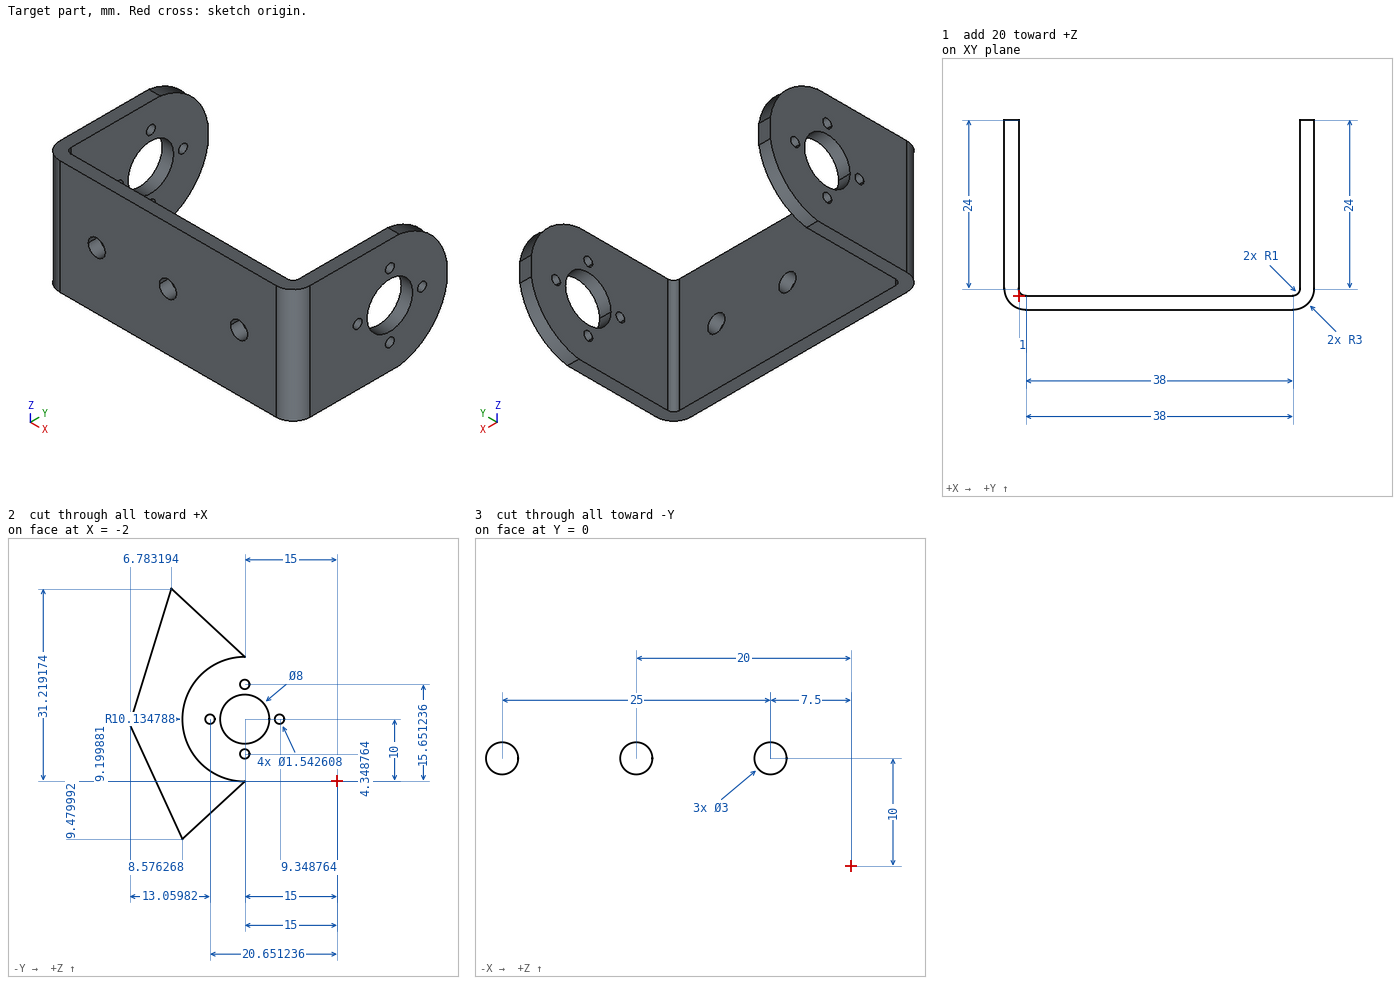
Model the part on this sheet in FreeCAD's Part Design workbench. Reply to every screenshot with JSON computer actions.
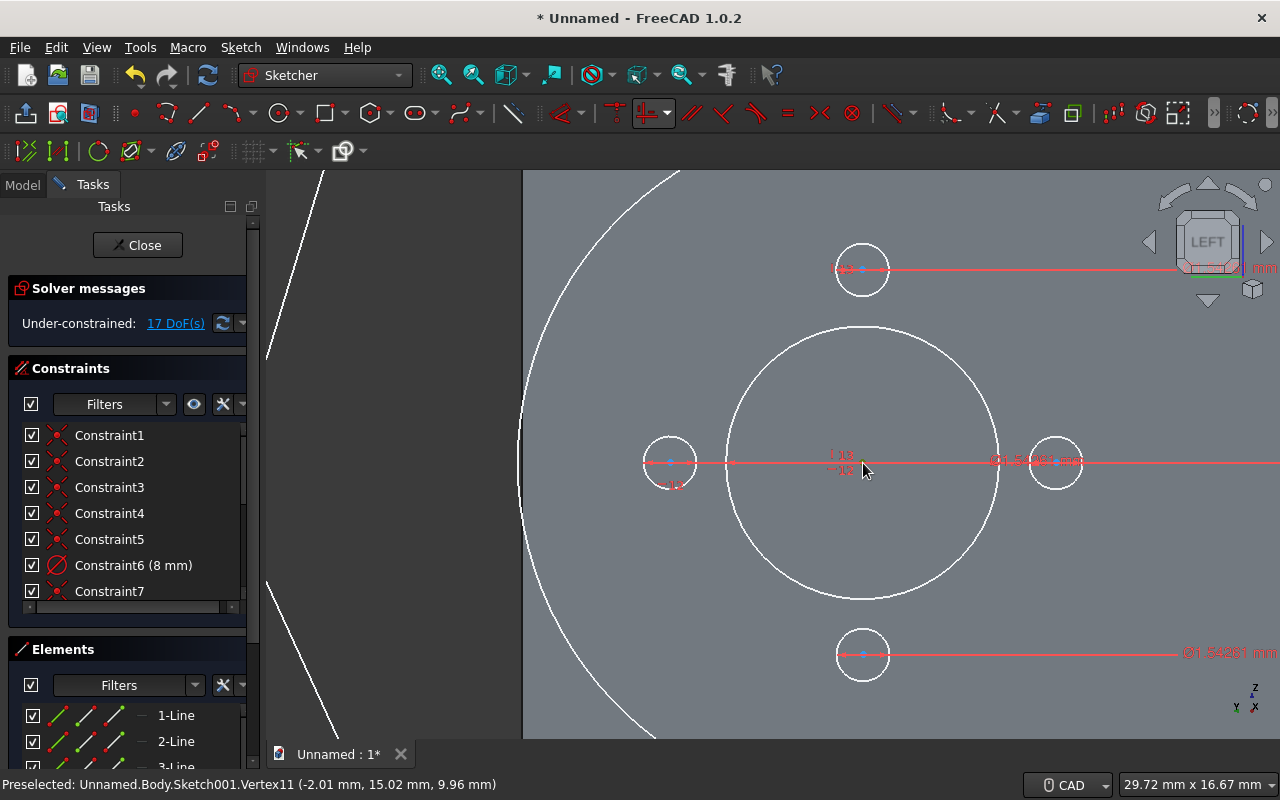
{"action": "left_click", "coordinate": [1056, 463]}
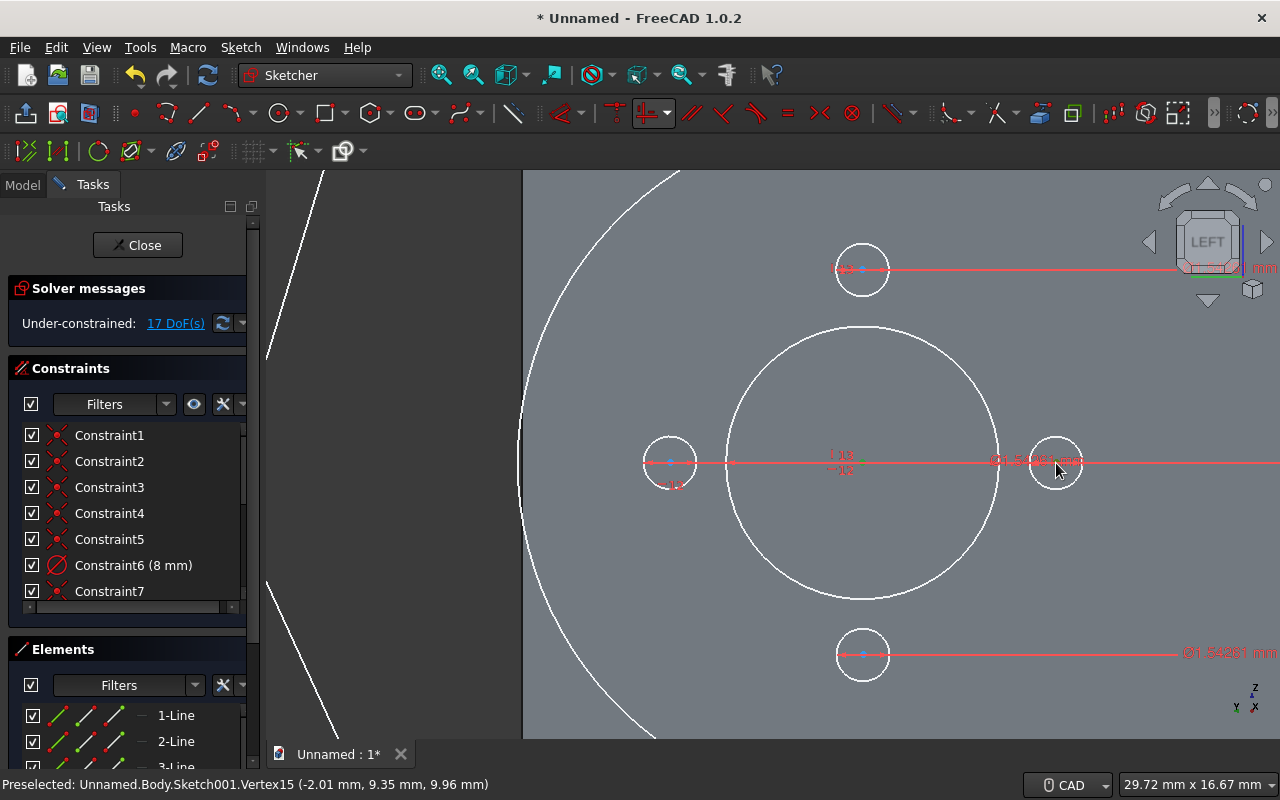
{"action": "left_click", "coordinate": [670, 114]}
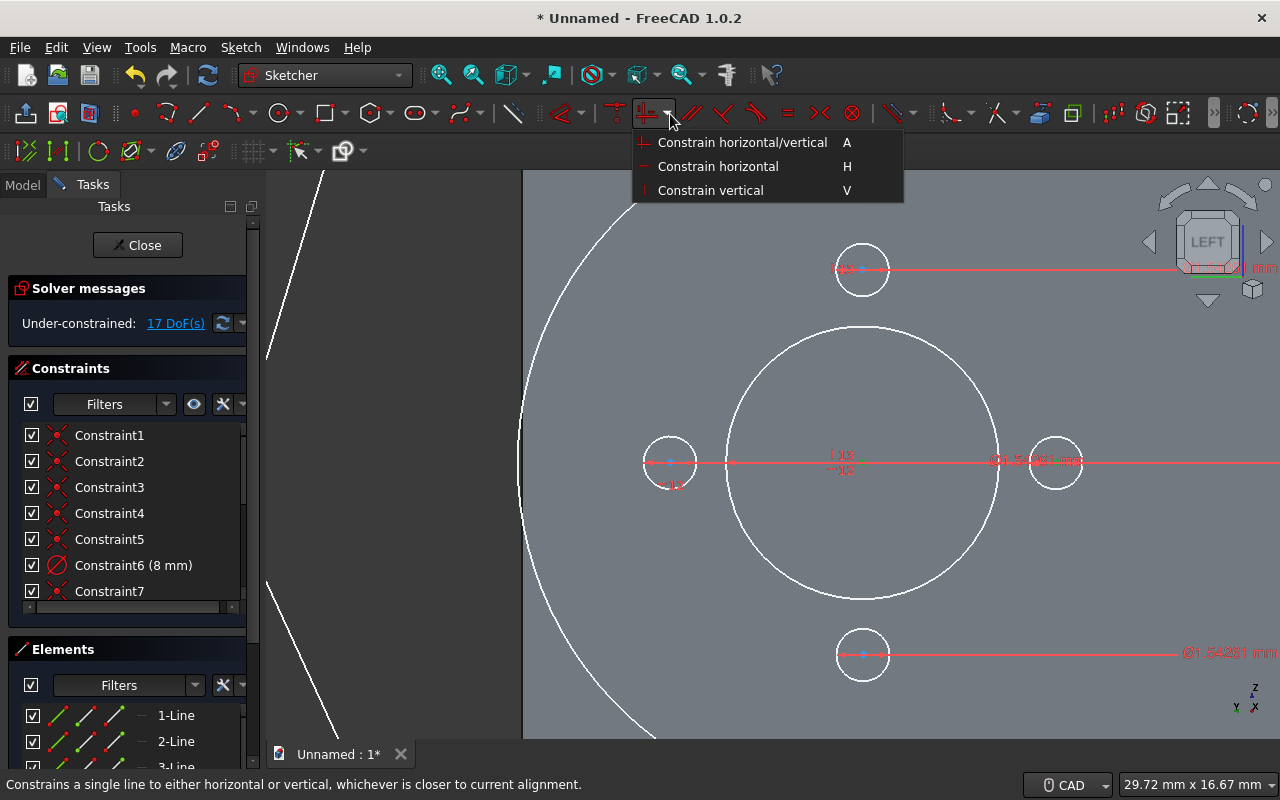
{"action": "left_click", "coordinate": [768, 166]}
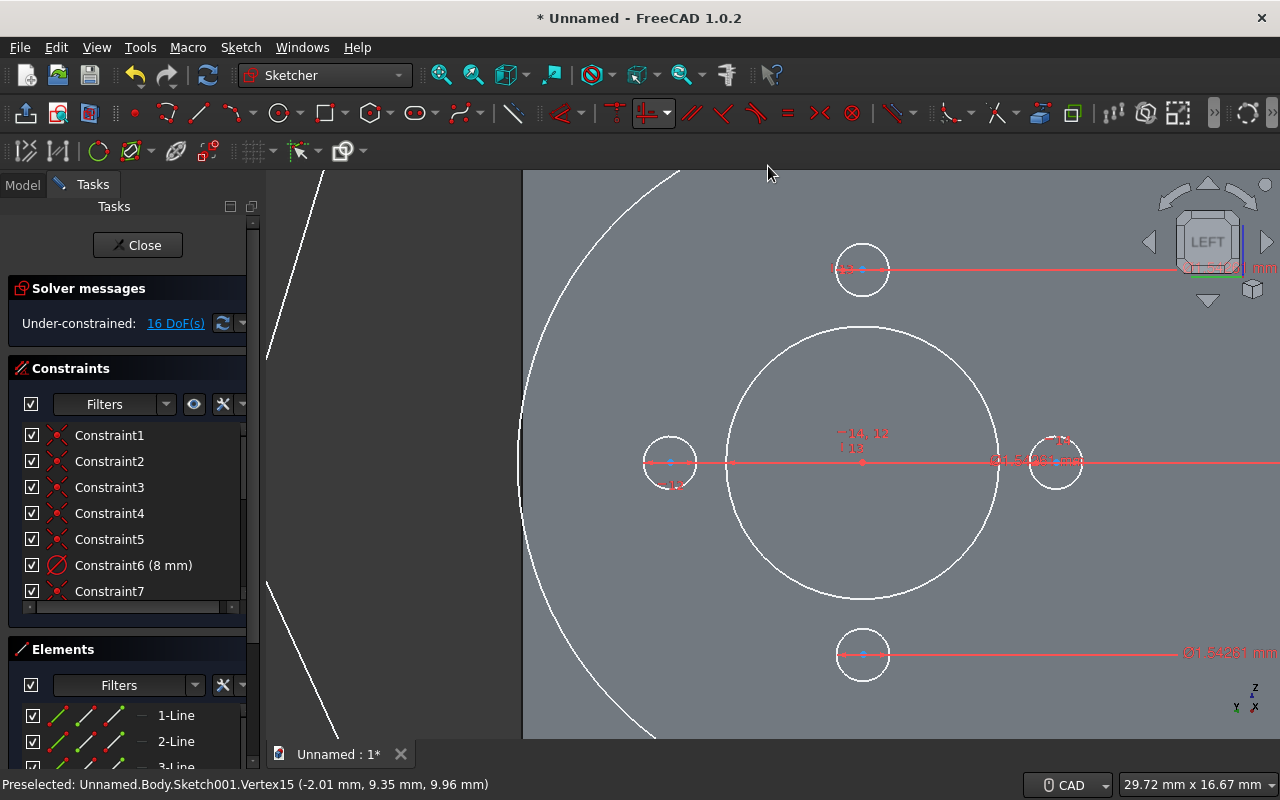
{"action": "left_click", "coordinate": [863, 463]}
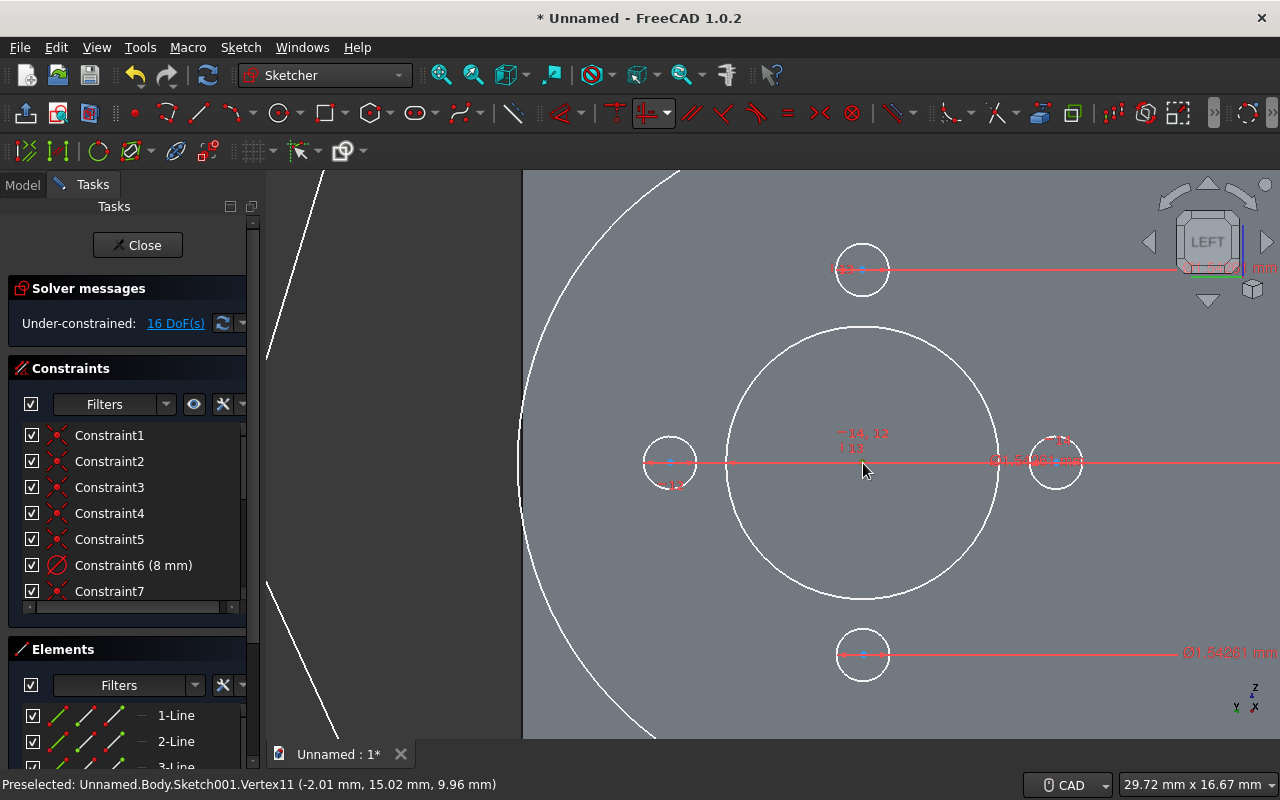
{"action": "left_click", "coordinate": [863, 655]}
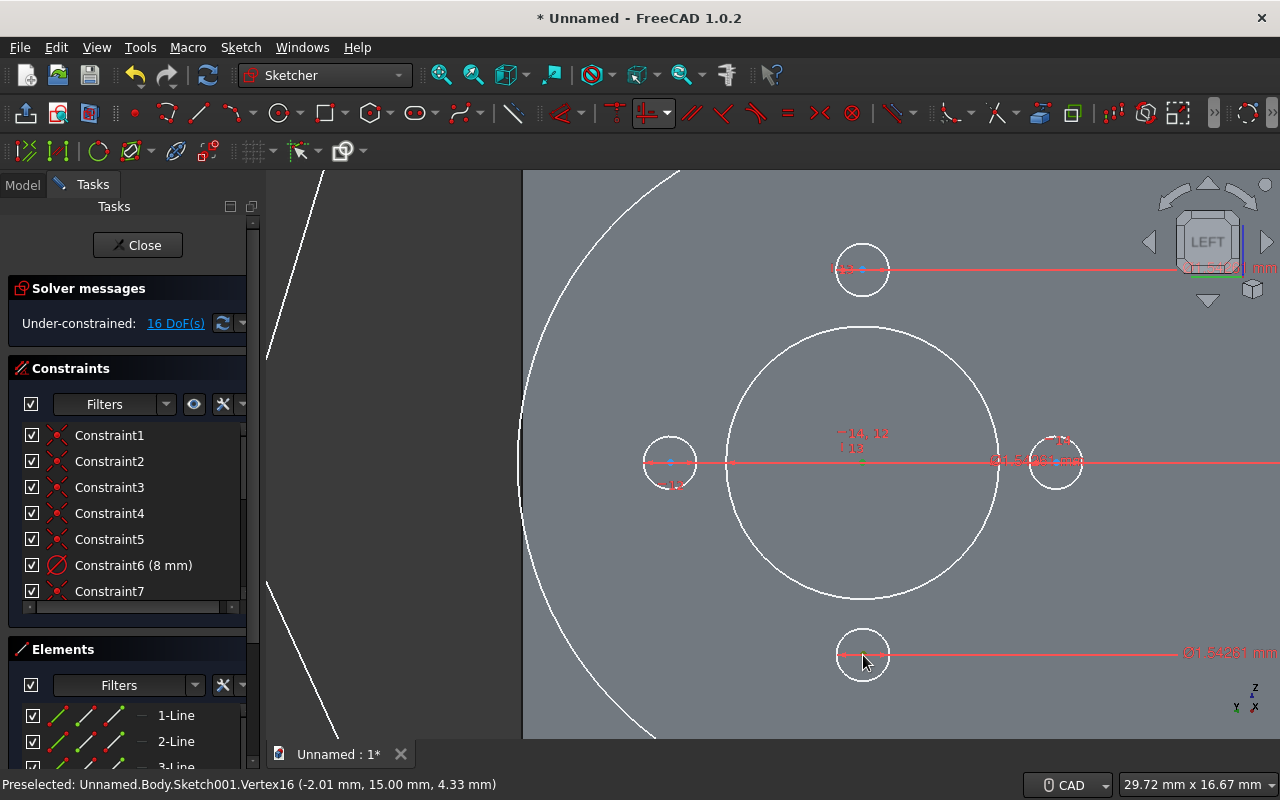
{"action": "left_click", "coordinate": [670, 114]}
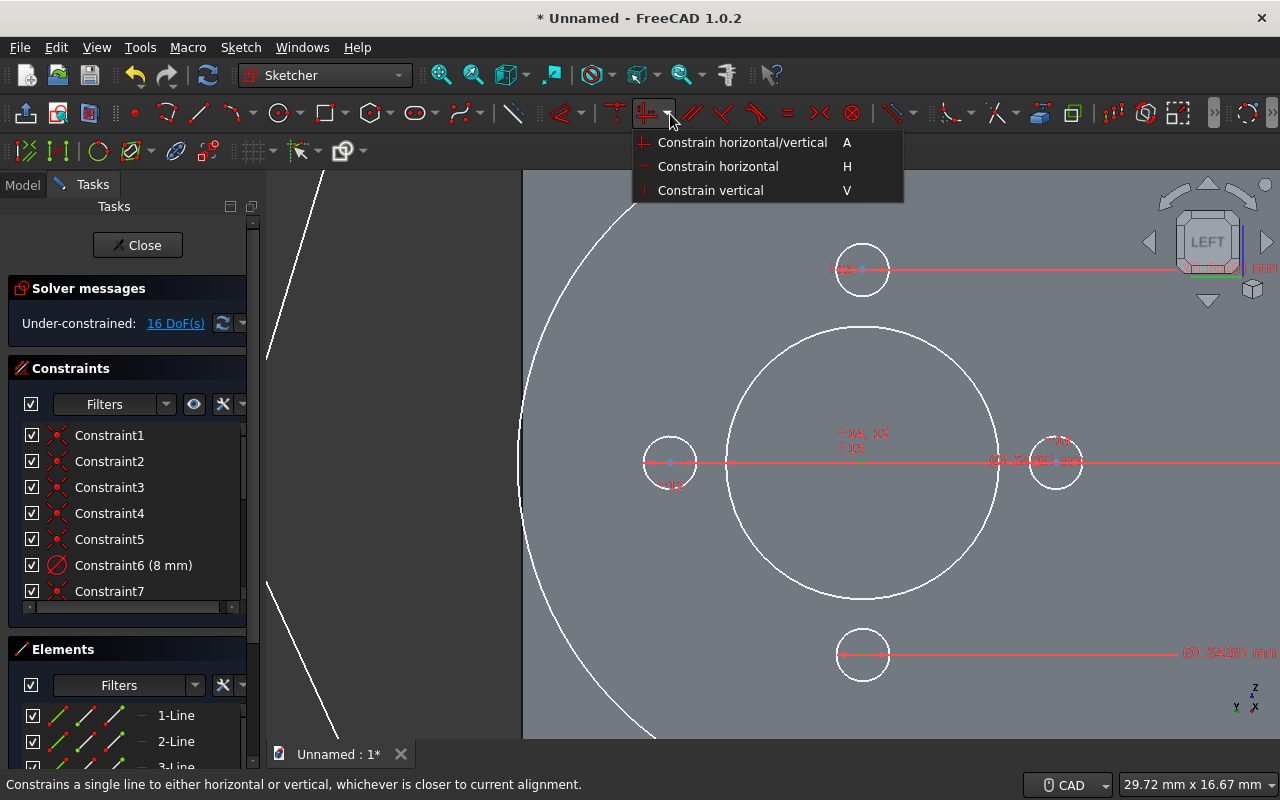
{"action": "left_click", "coordinate": [768, 190]}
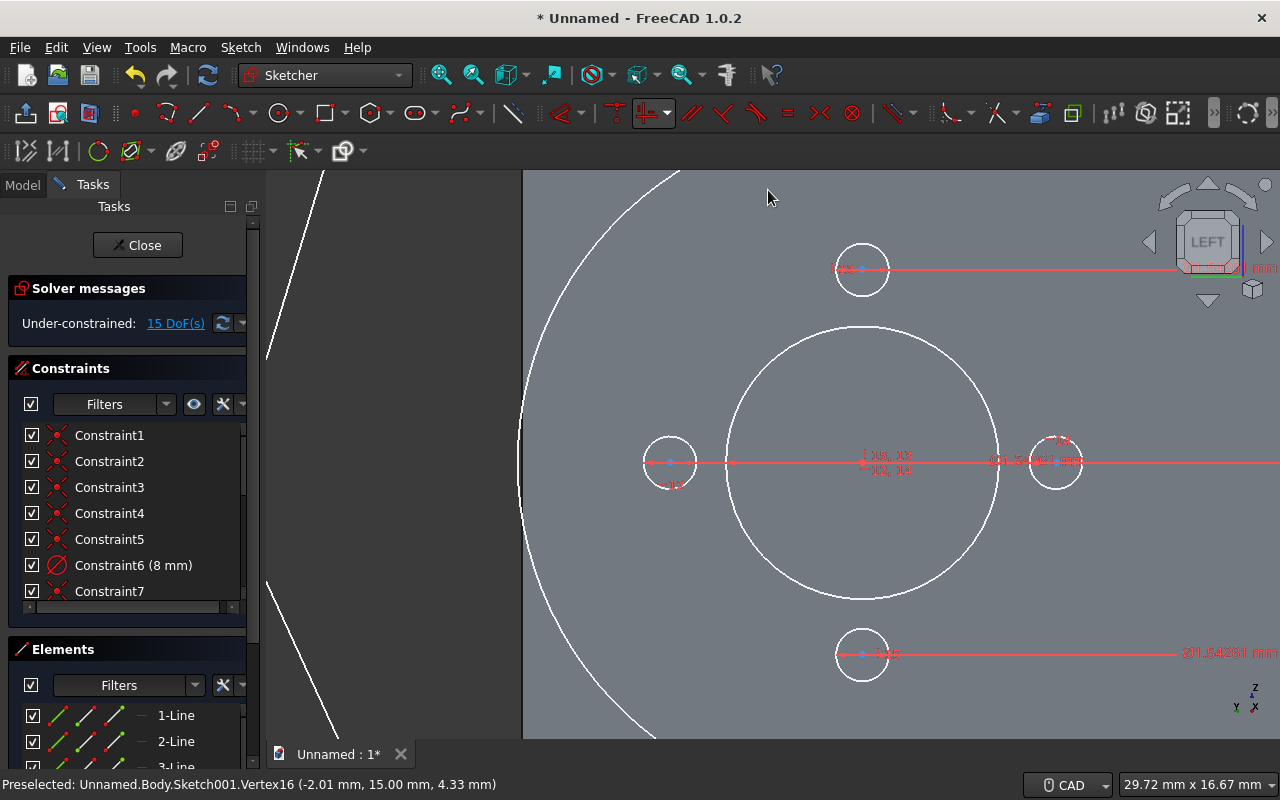
{"action": "left_click", "coordinate": [560, 114]}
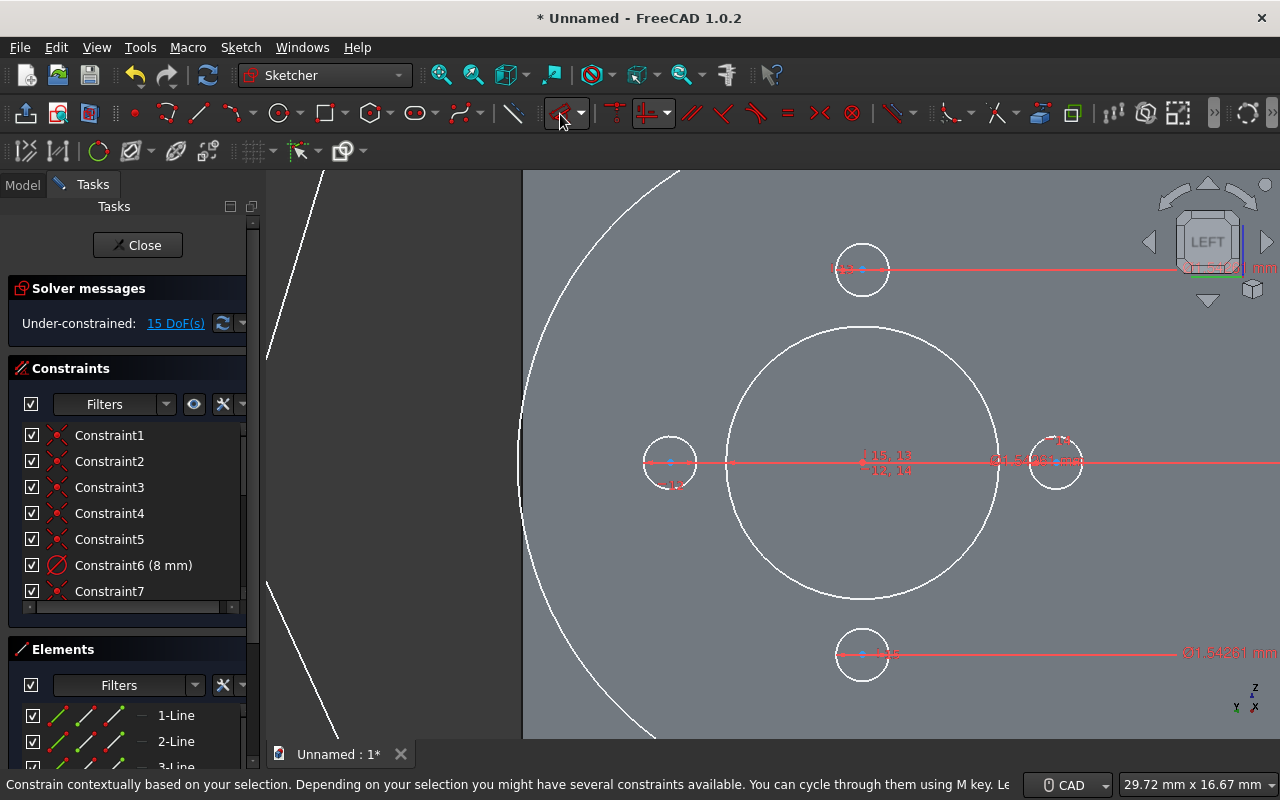
{"action": "left_click", "coordinate": [584, 260]}
{"action": "left_click", "coordinate": [558, 241]}